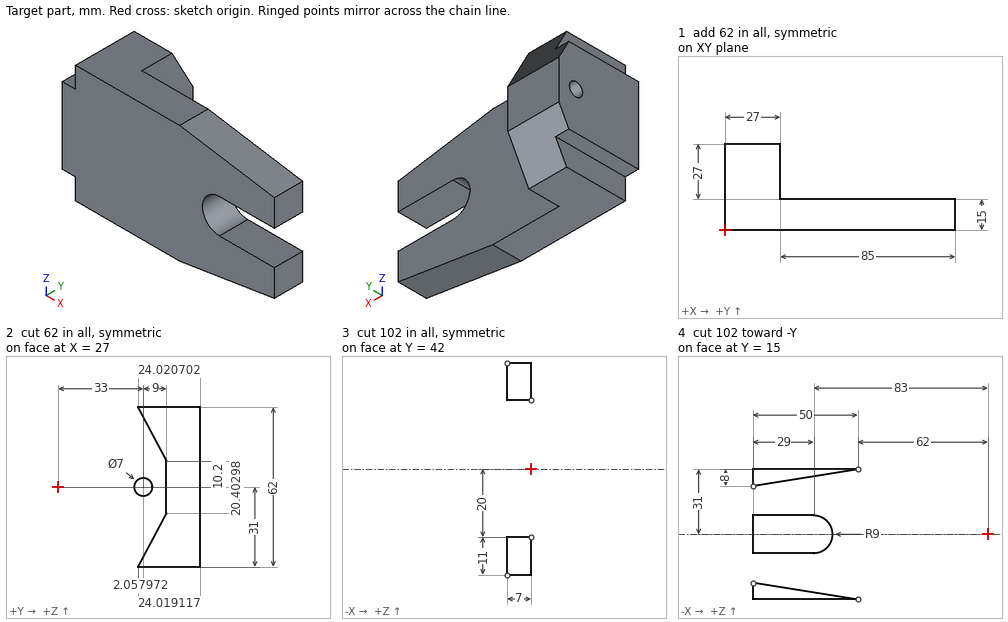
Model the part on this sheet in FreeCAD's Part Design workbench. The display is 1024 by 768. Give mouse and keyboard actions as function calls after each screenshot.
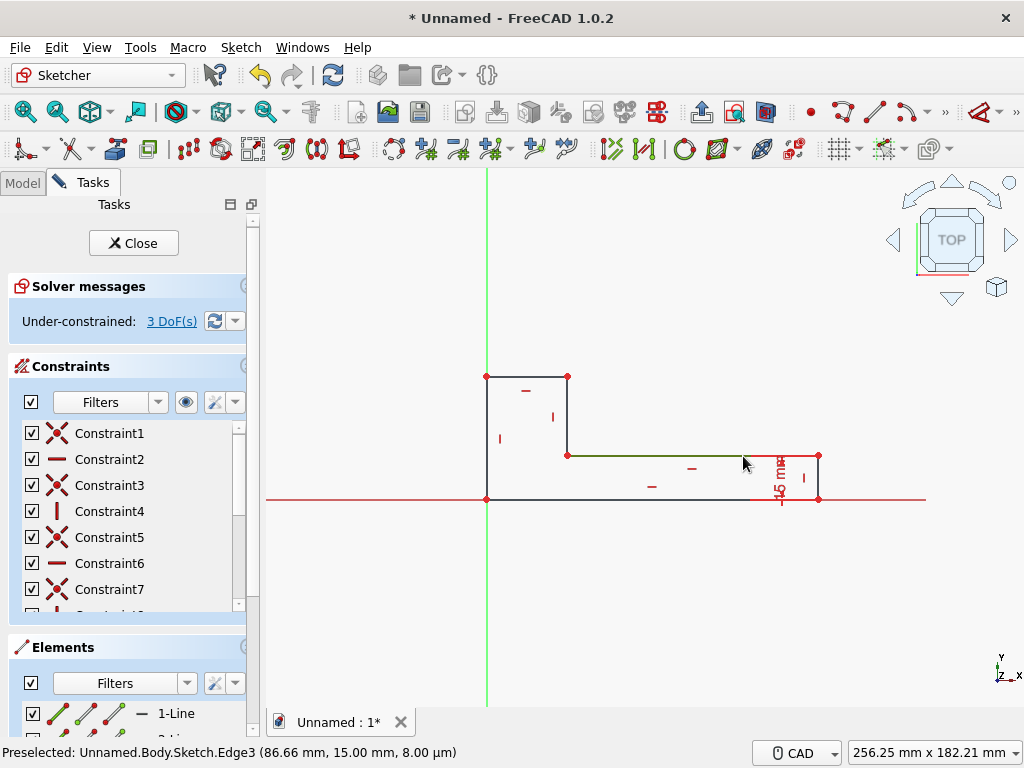
click(1002, 112)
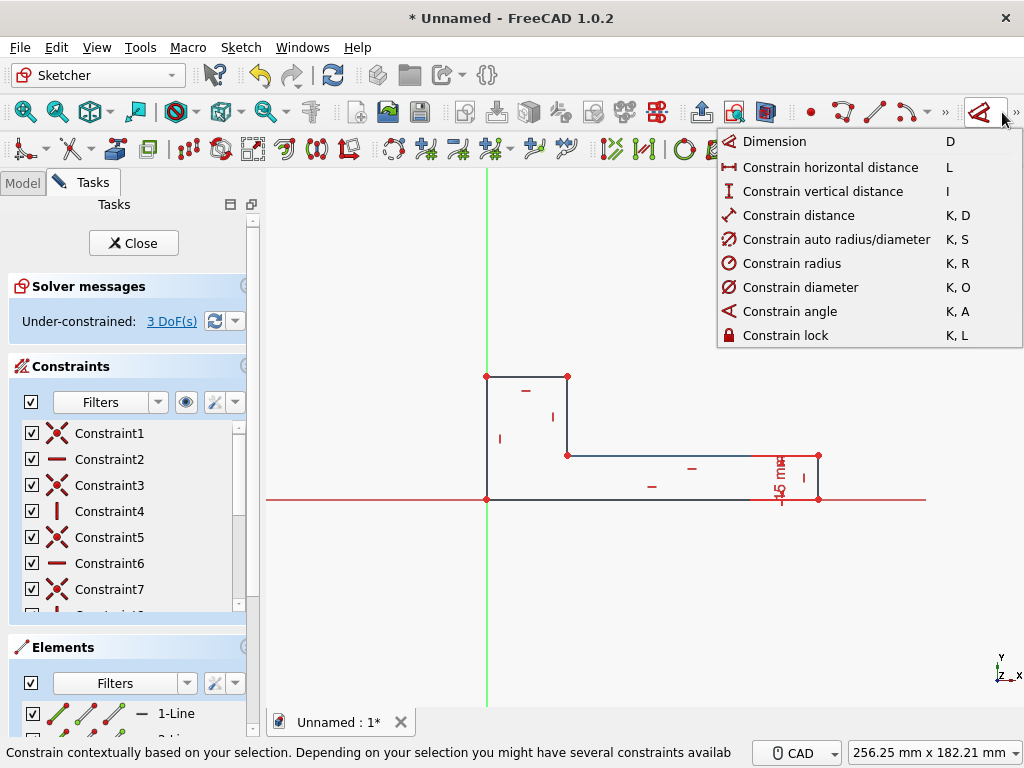
click(870, 167)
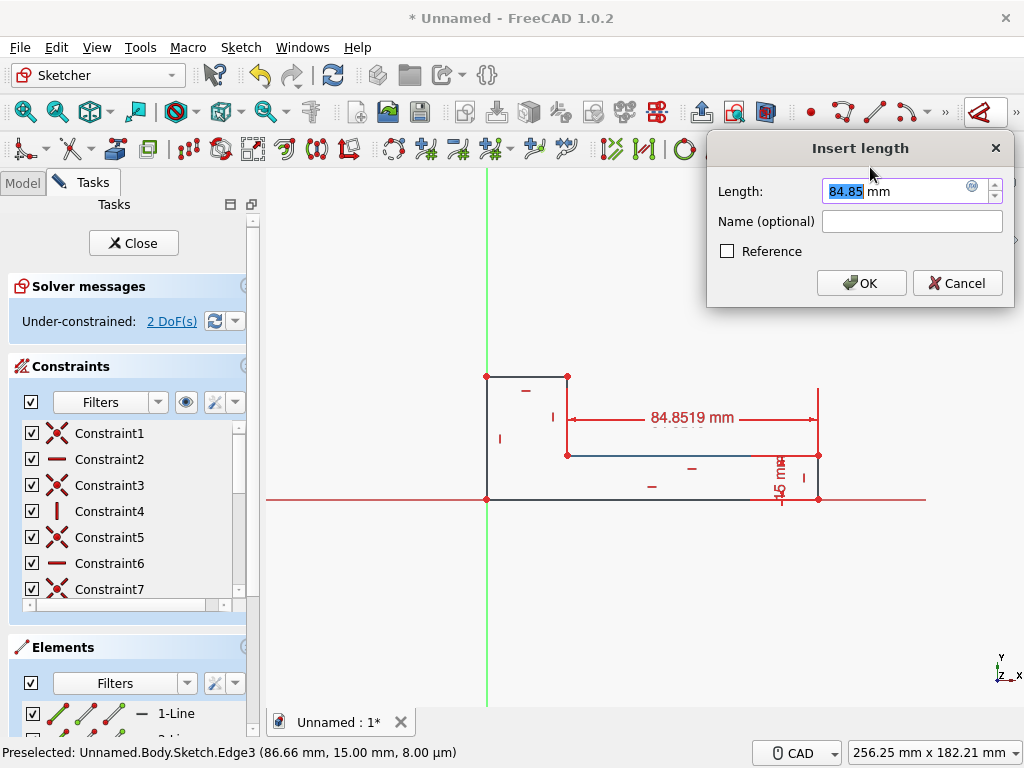
text(85)
key(Return)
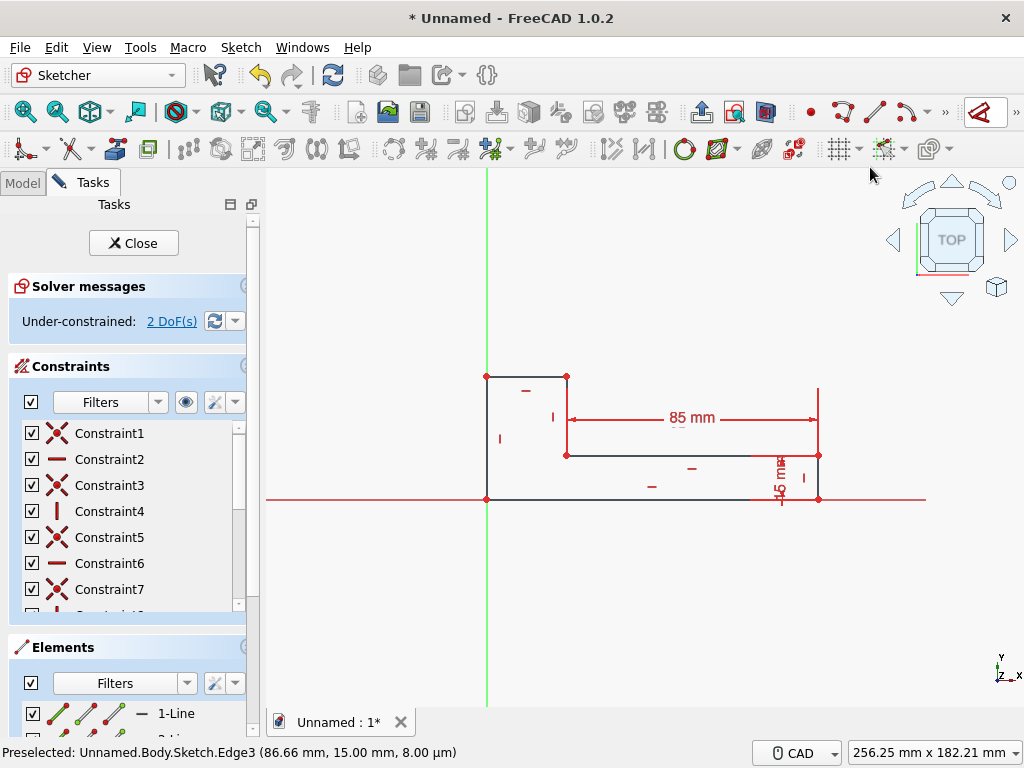
click(567, 432)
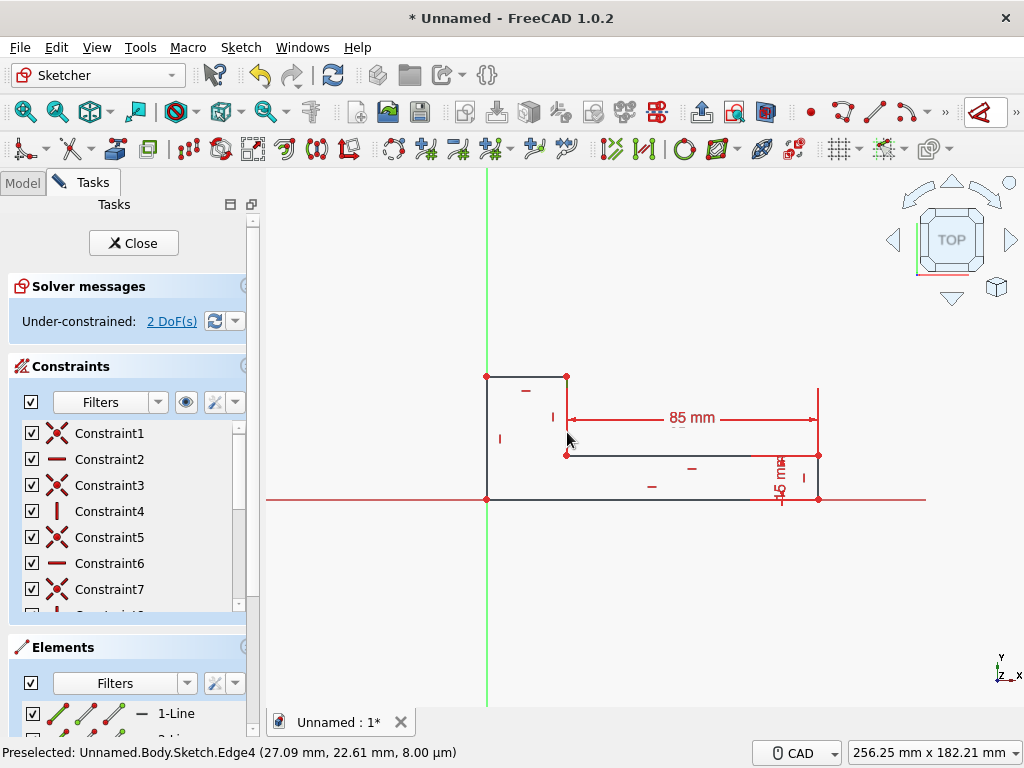
key(i)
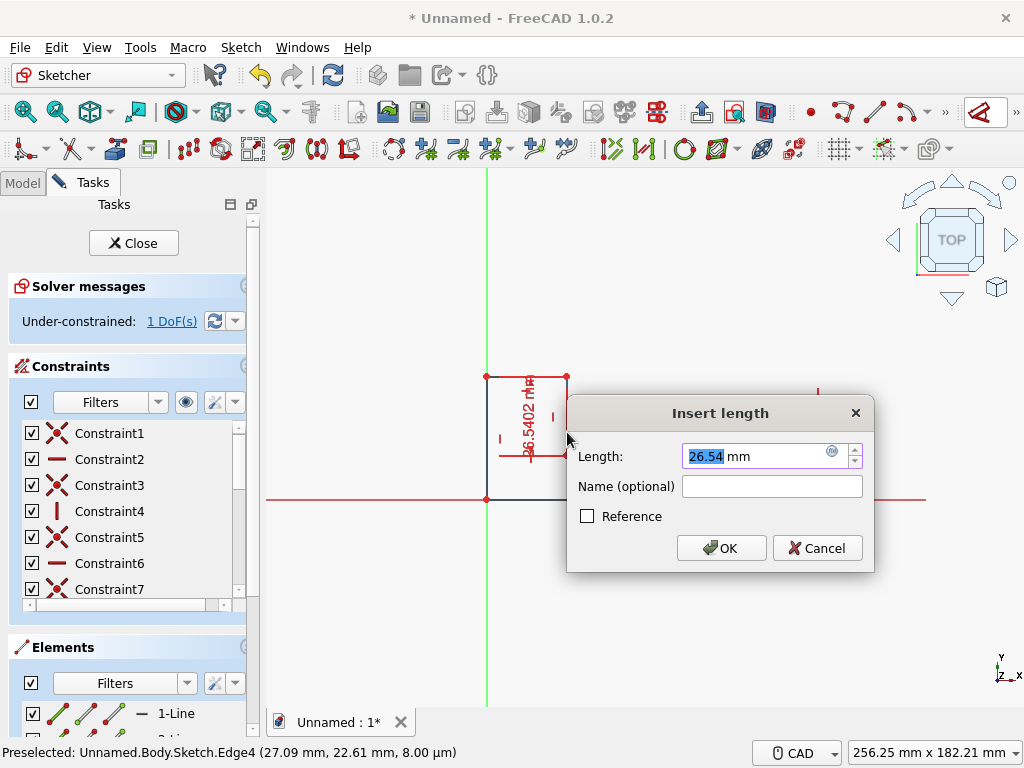
text(27)
key(Return)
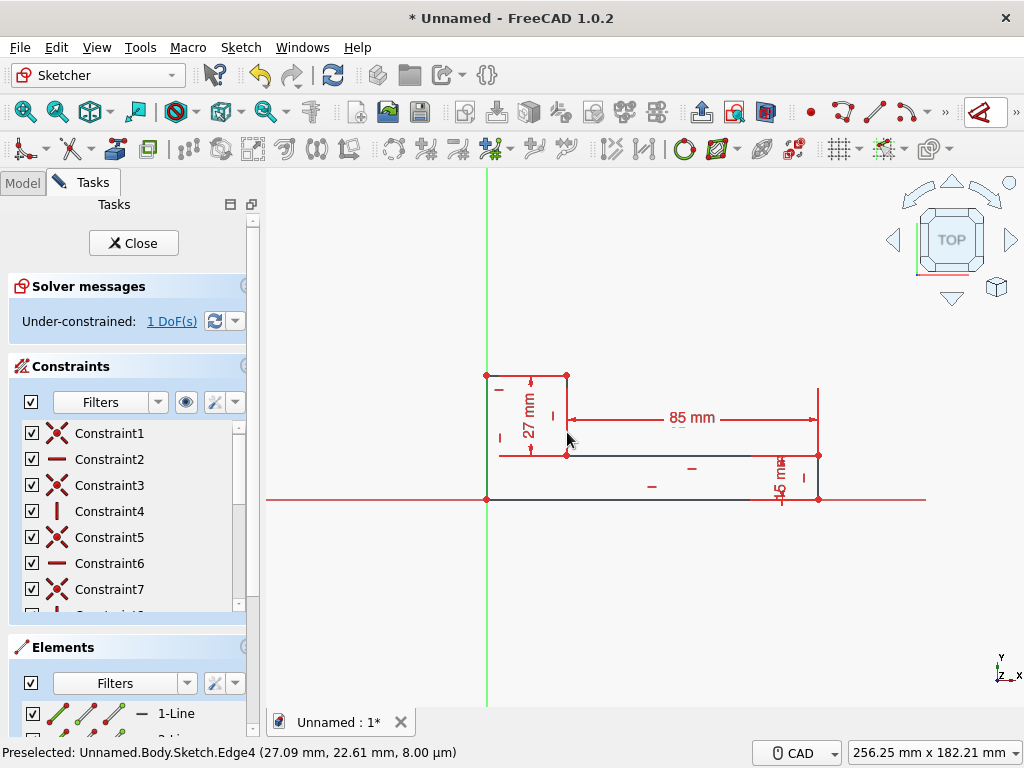
click(543, 376)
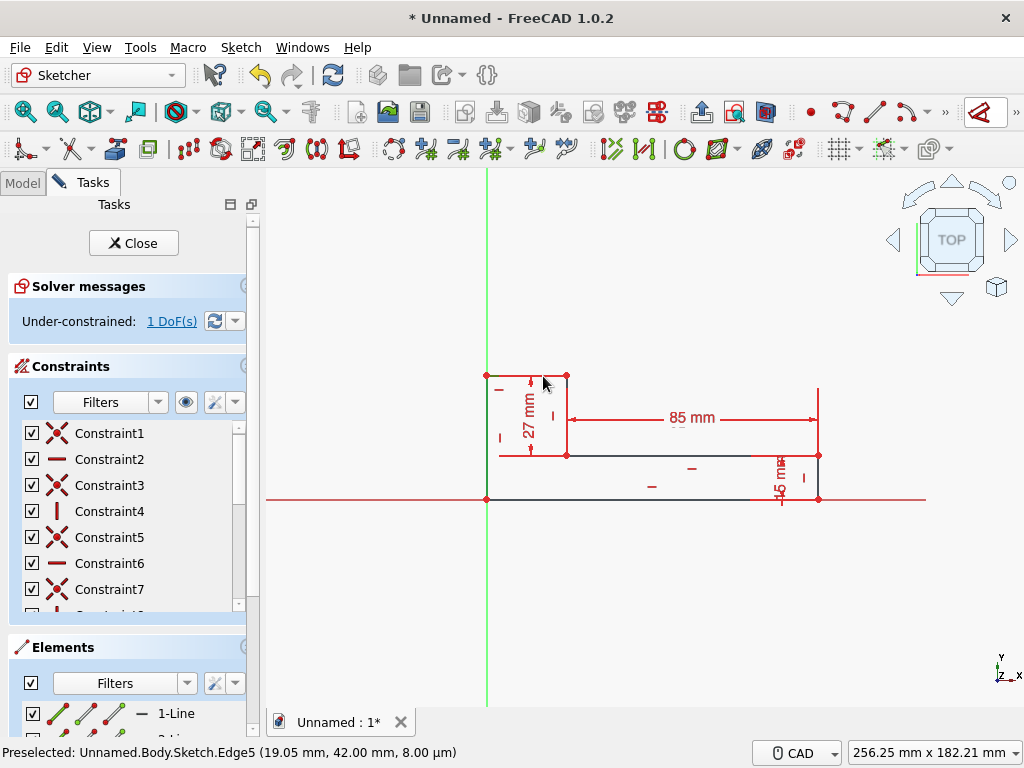
key(l)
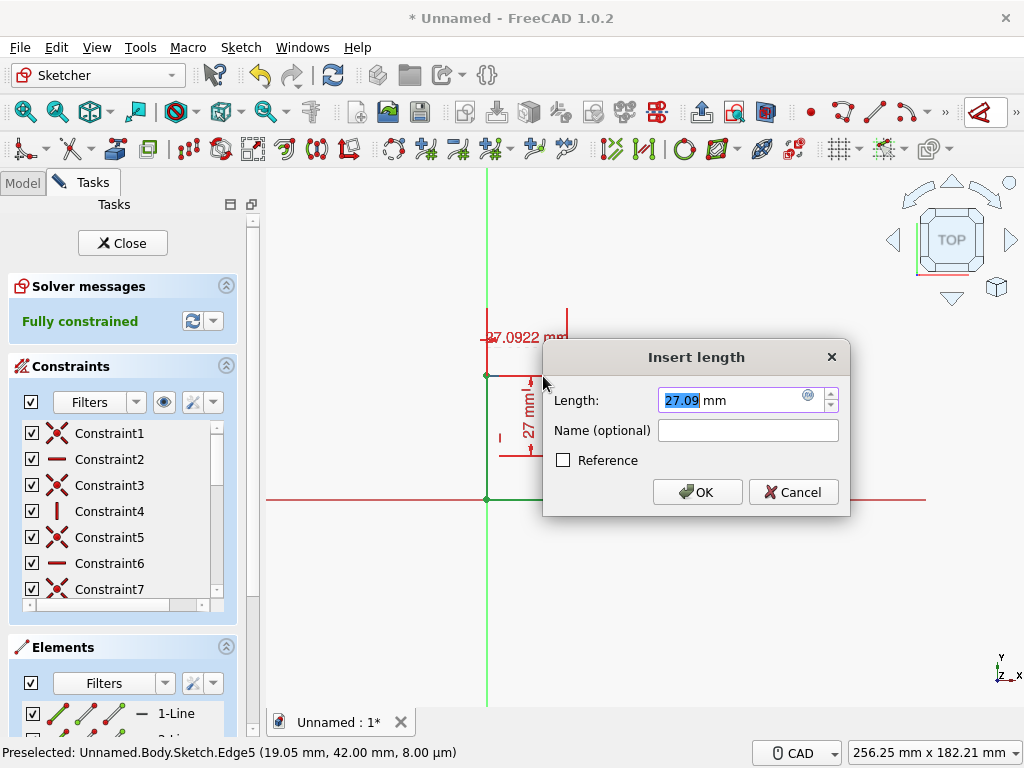
text(27)
key(Return)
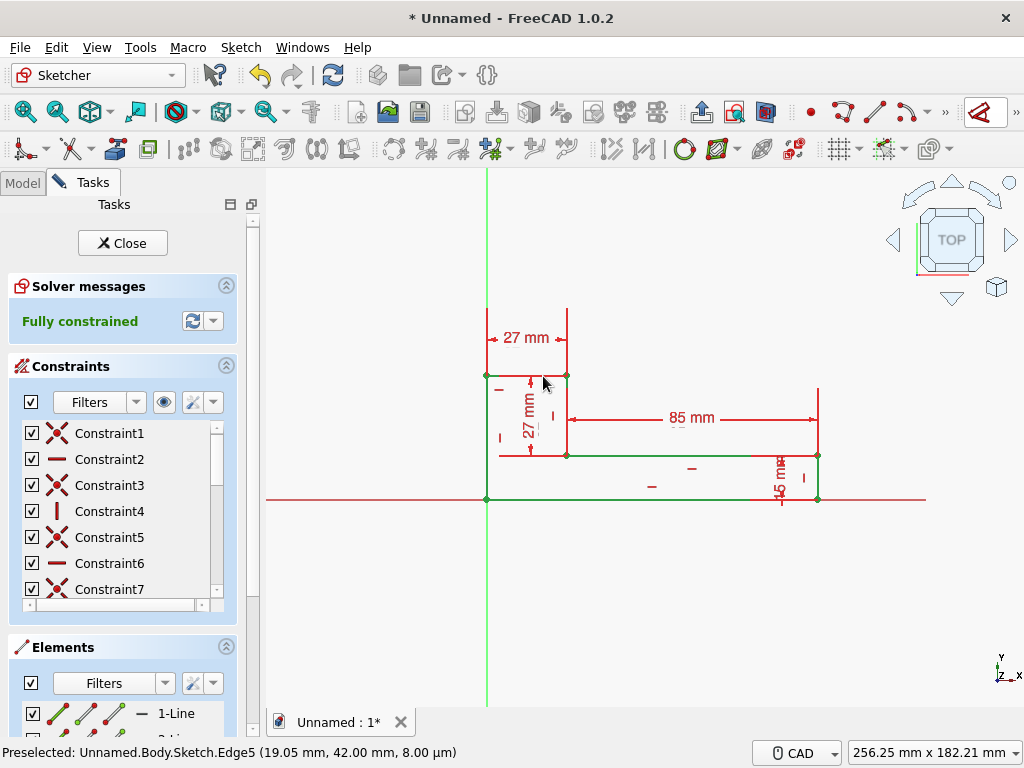
click(123, 243)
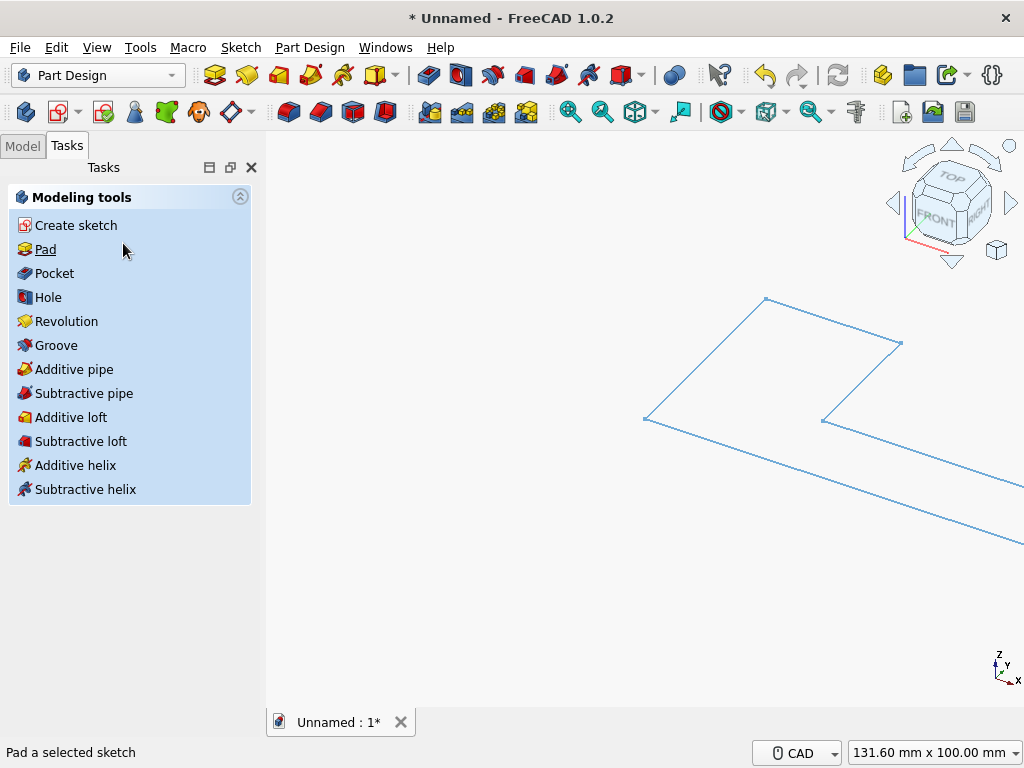
click(216, 76)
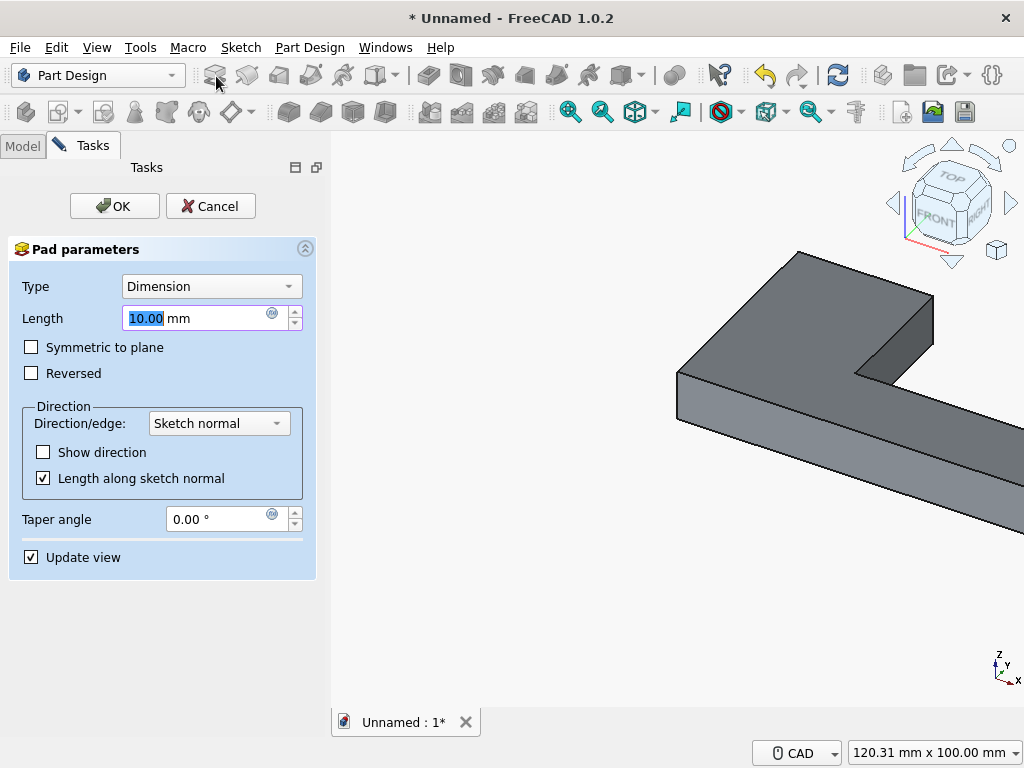
text(62)
key(Tab)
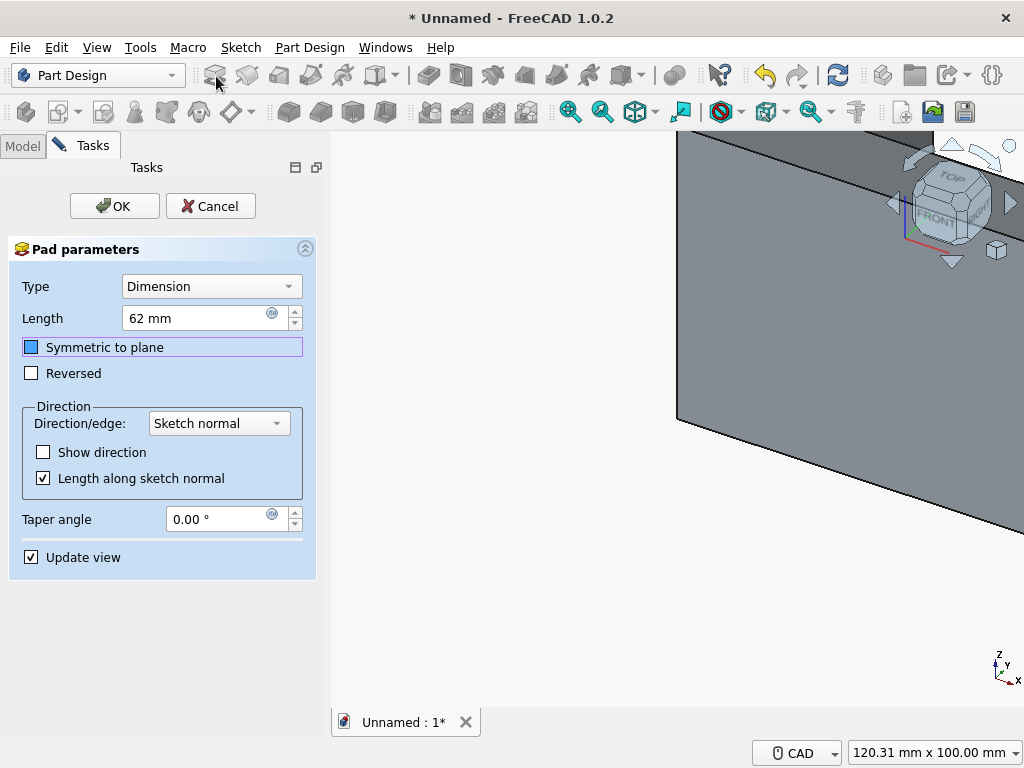
click(30, 347)